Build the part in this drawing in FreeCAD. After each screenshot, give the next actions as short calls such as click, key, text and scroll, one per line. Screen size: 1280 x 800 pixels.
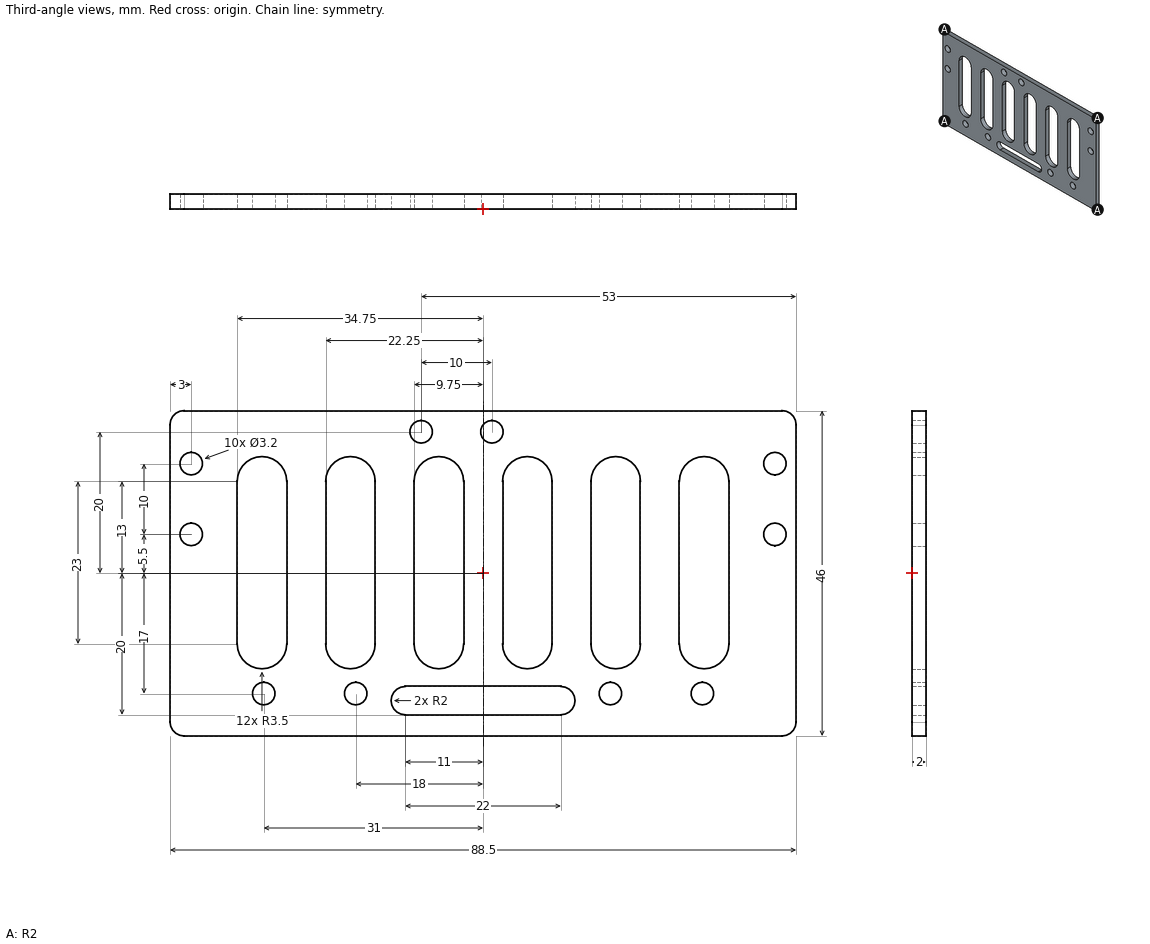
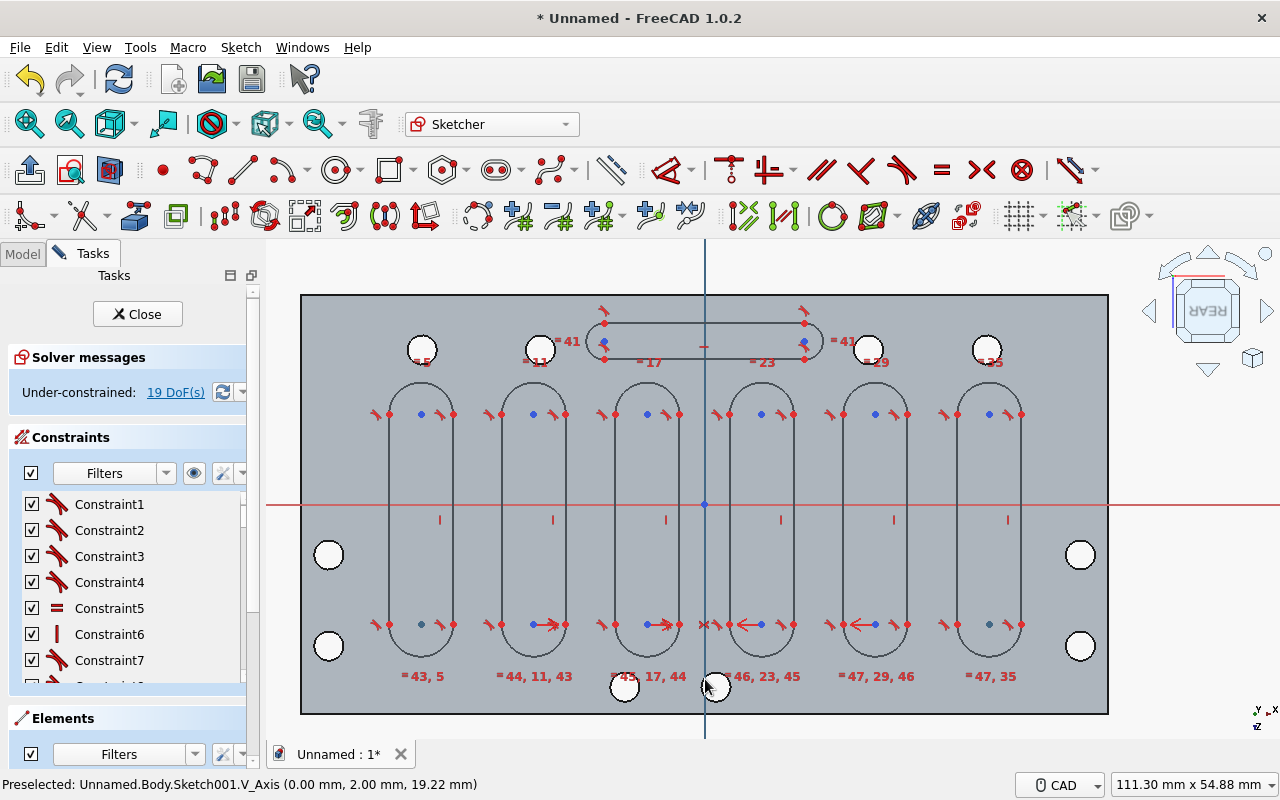
click(982, 170)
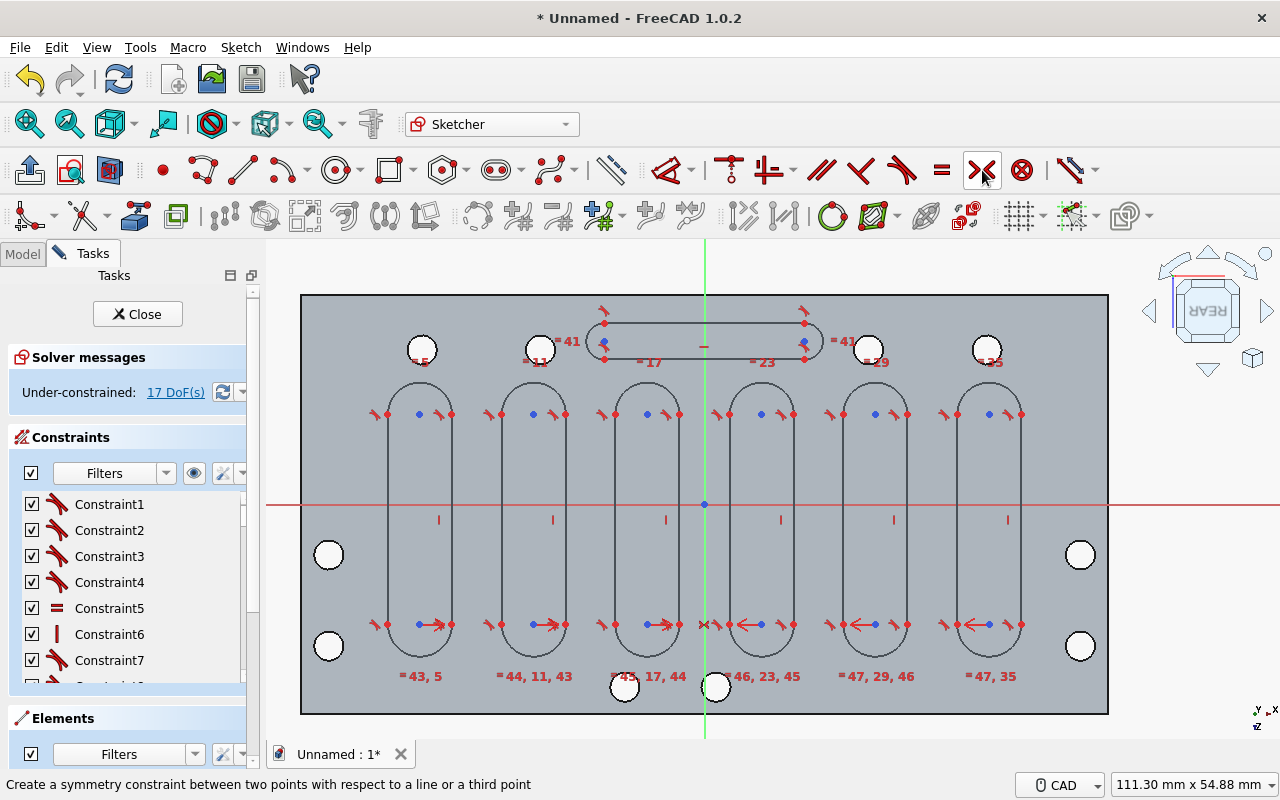
click(666, 170)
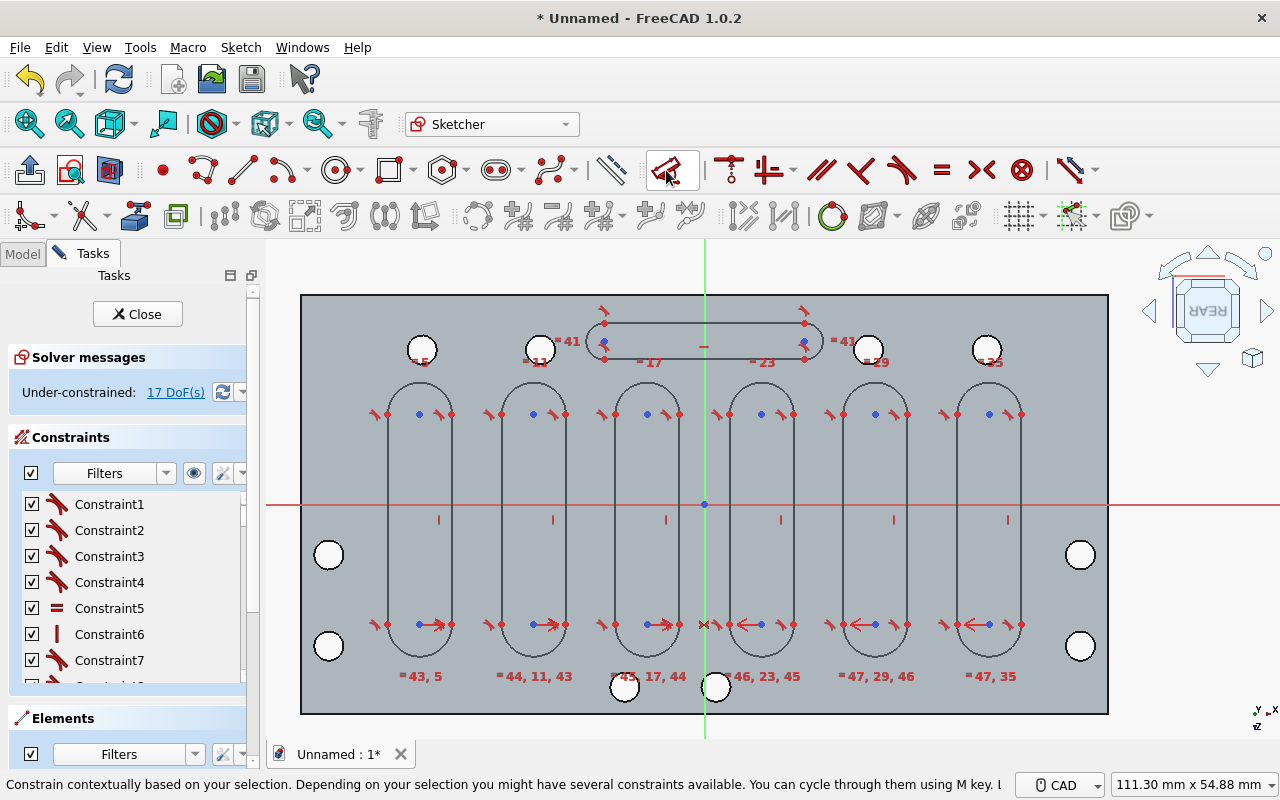
scroll(401, 651, up, 2)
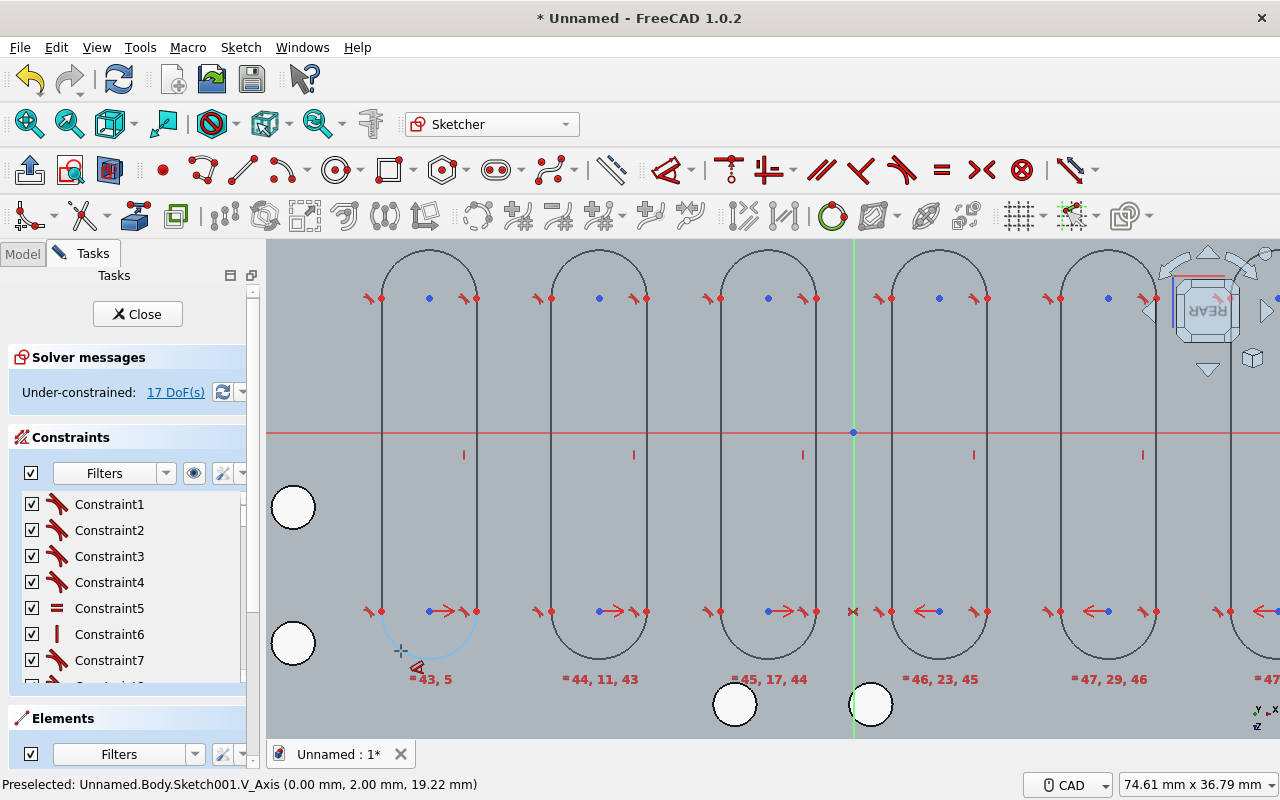
click(401, 650)
click(382, 676)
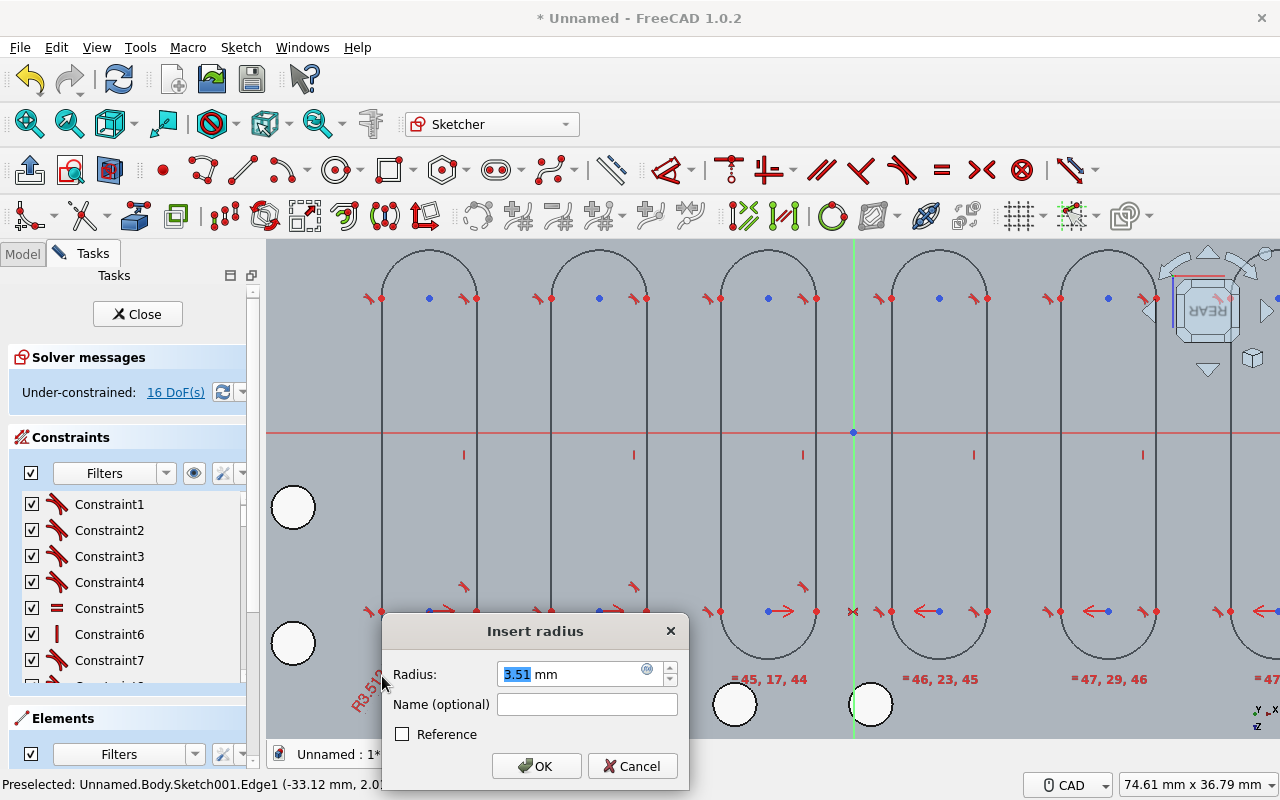
text(3.5)
key(Return)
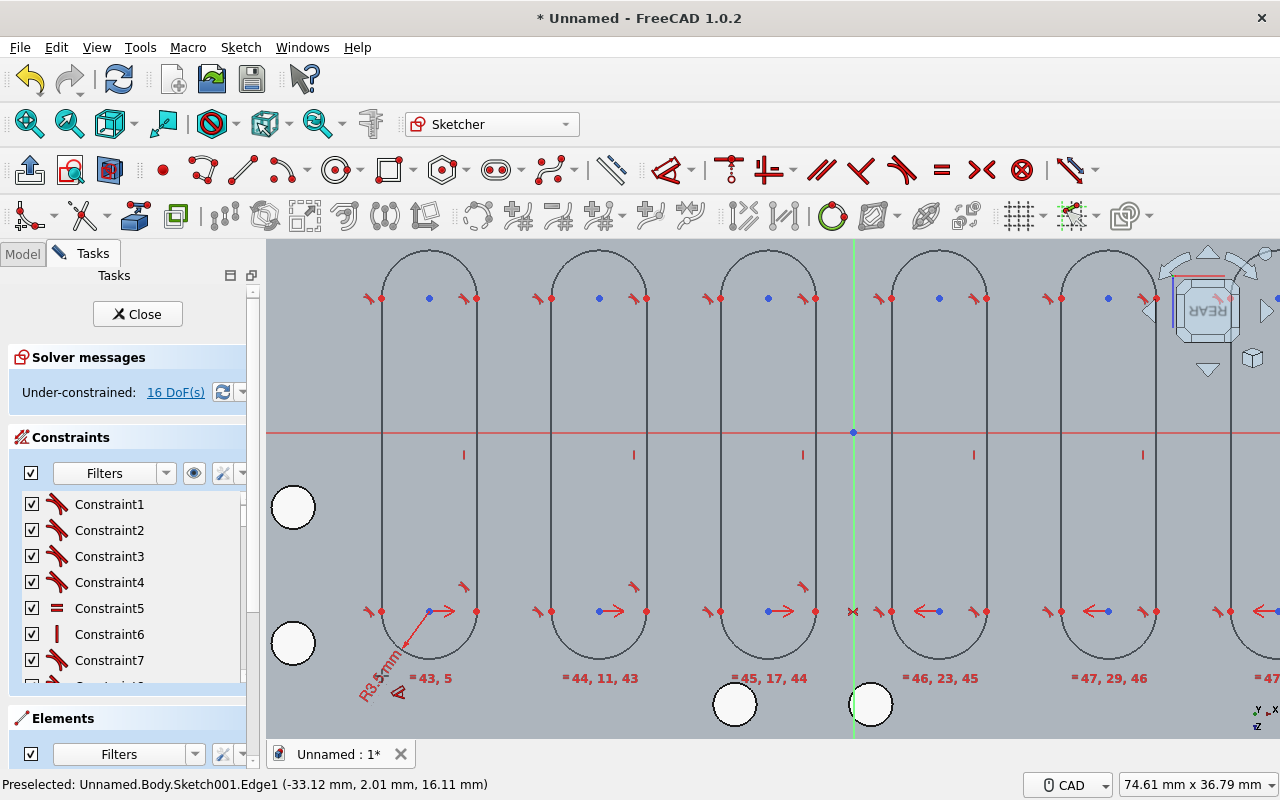
scroll(401, 652, down, 2)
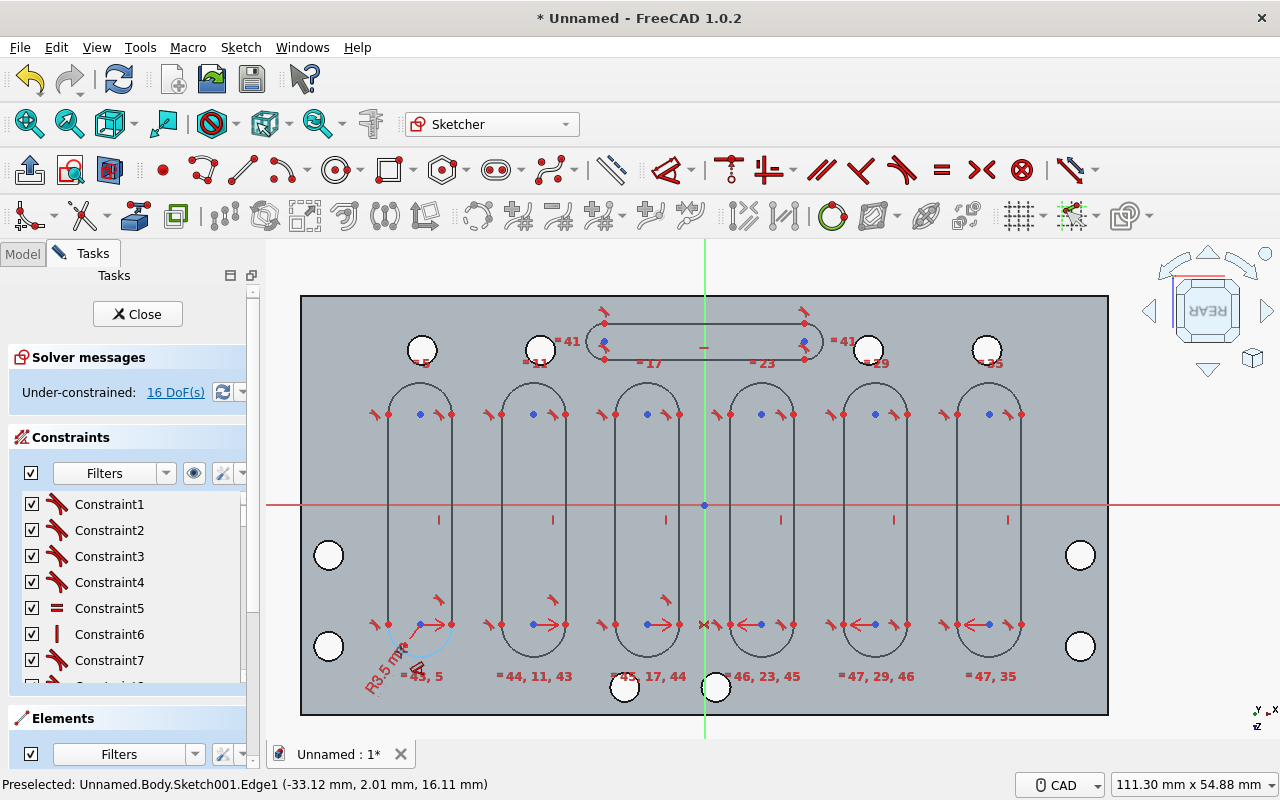
scroll(590, 331, up, 4)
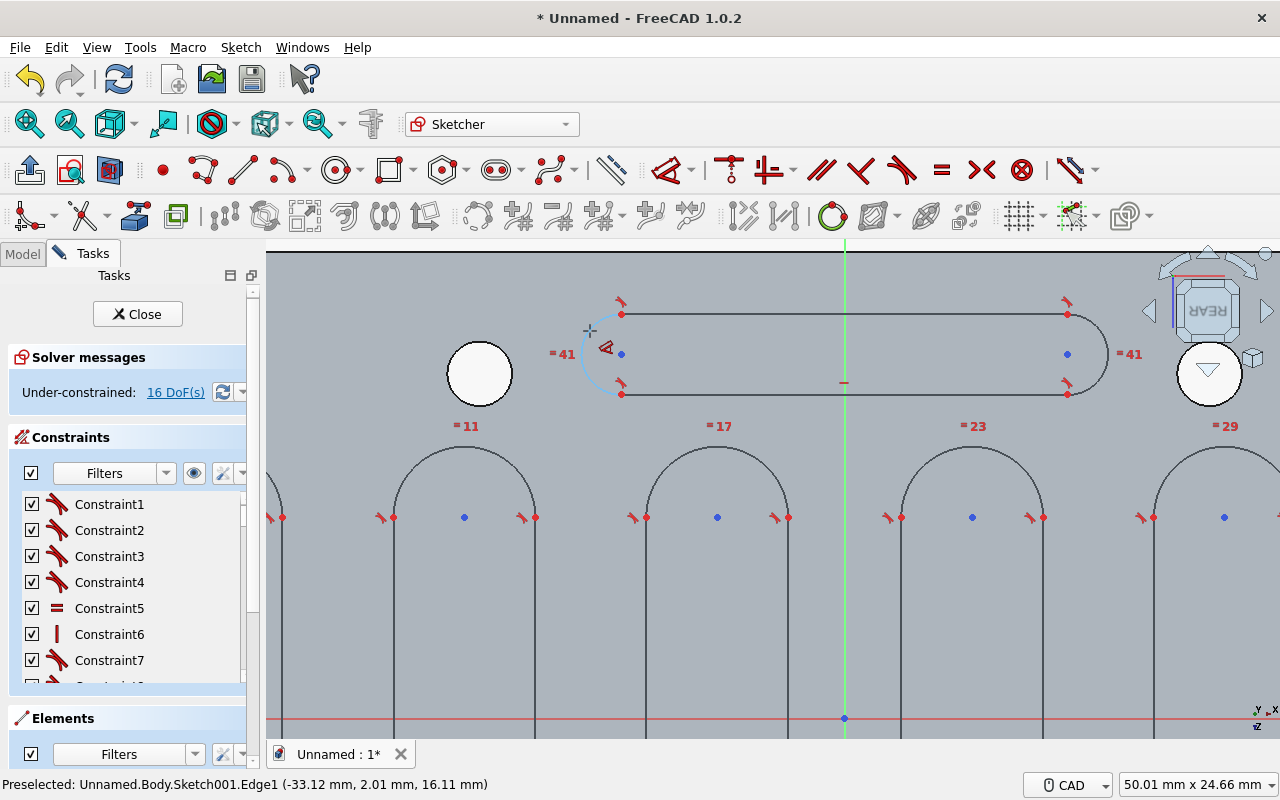
click(589, 331)
click(563, 312)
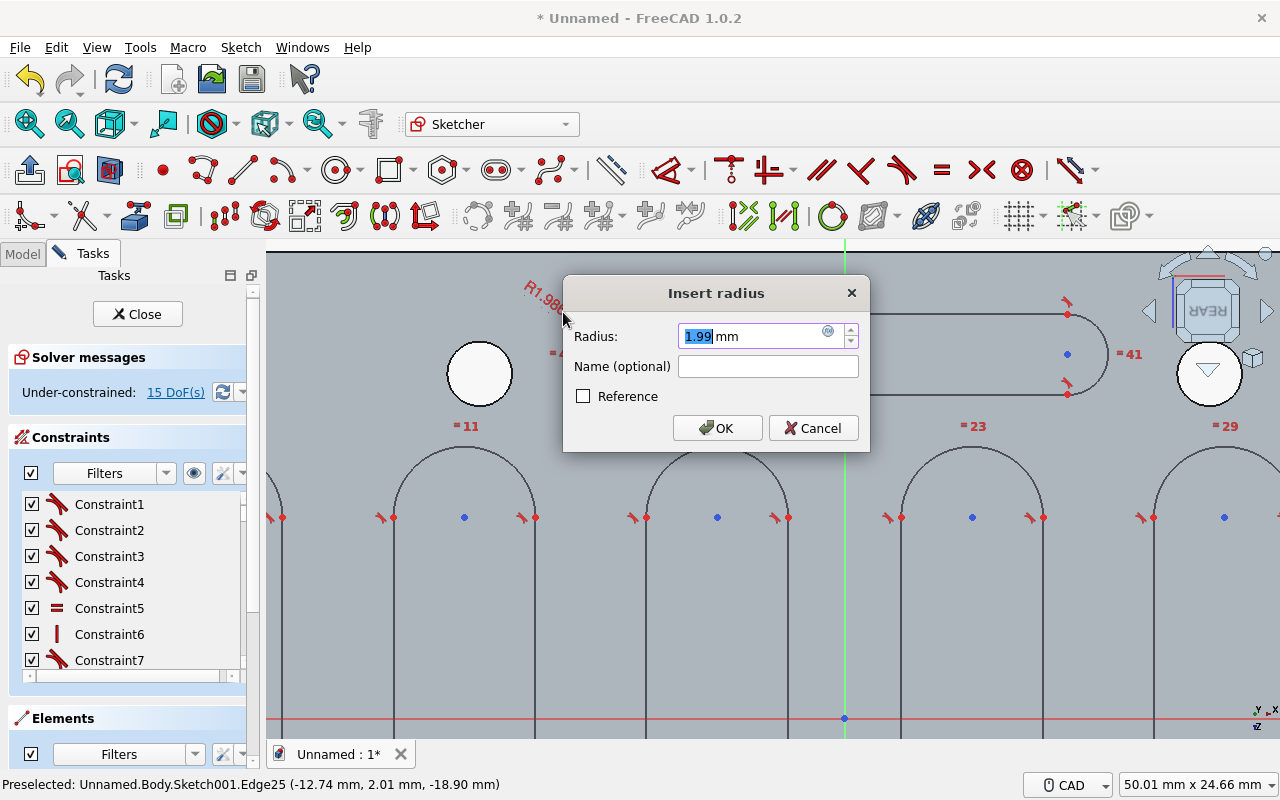
text(2)
key(Return)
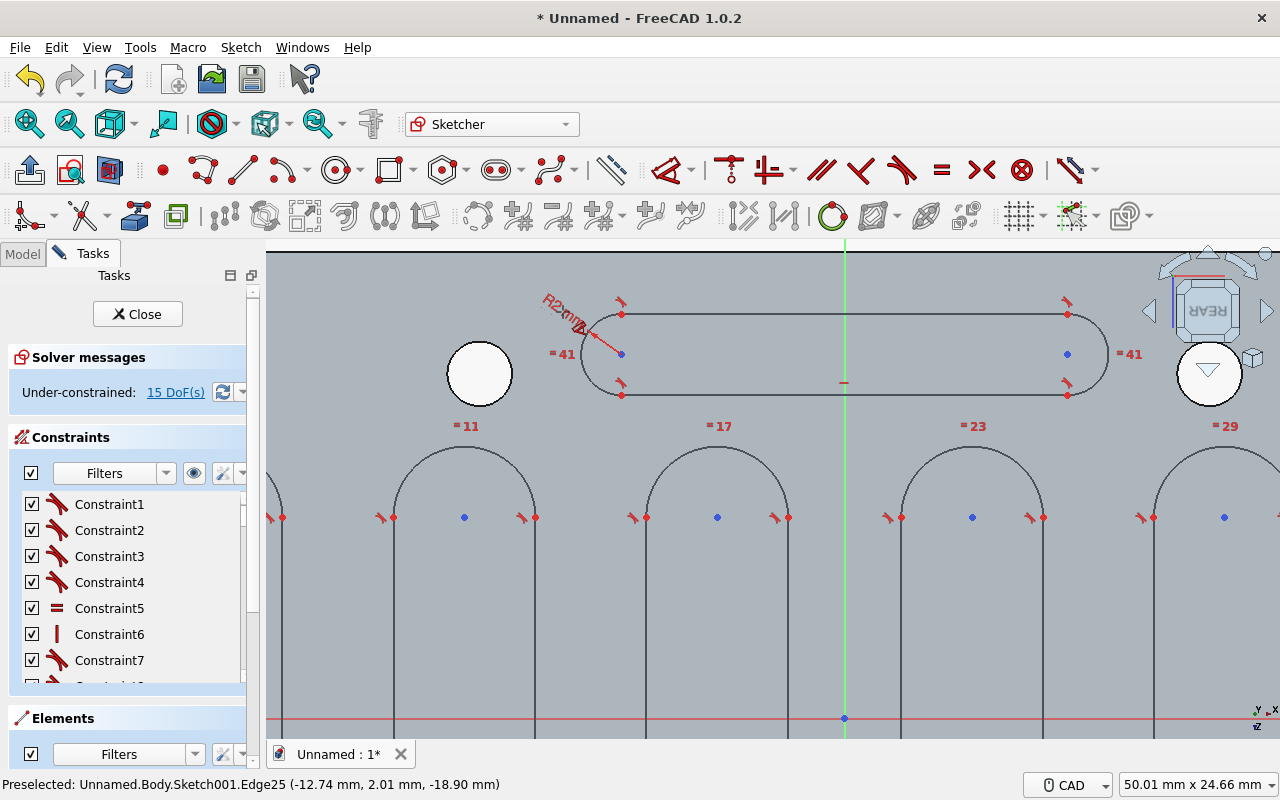
scroll(590, 331, down, 4)